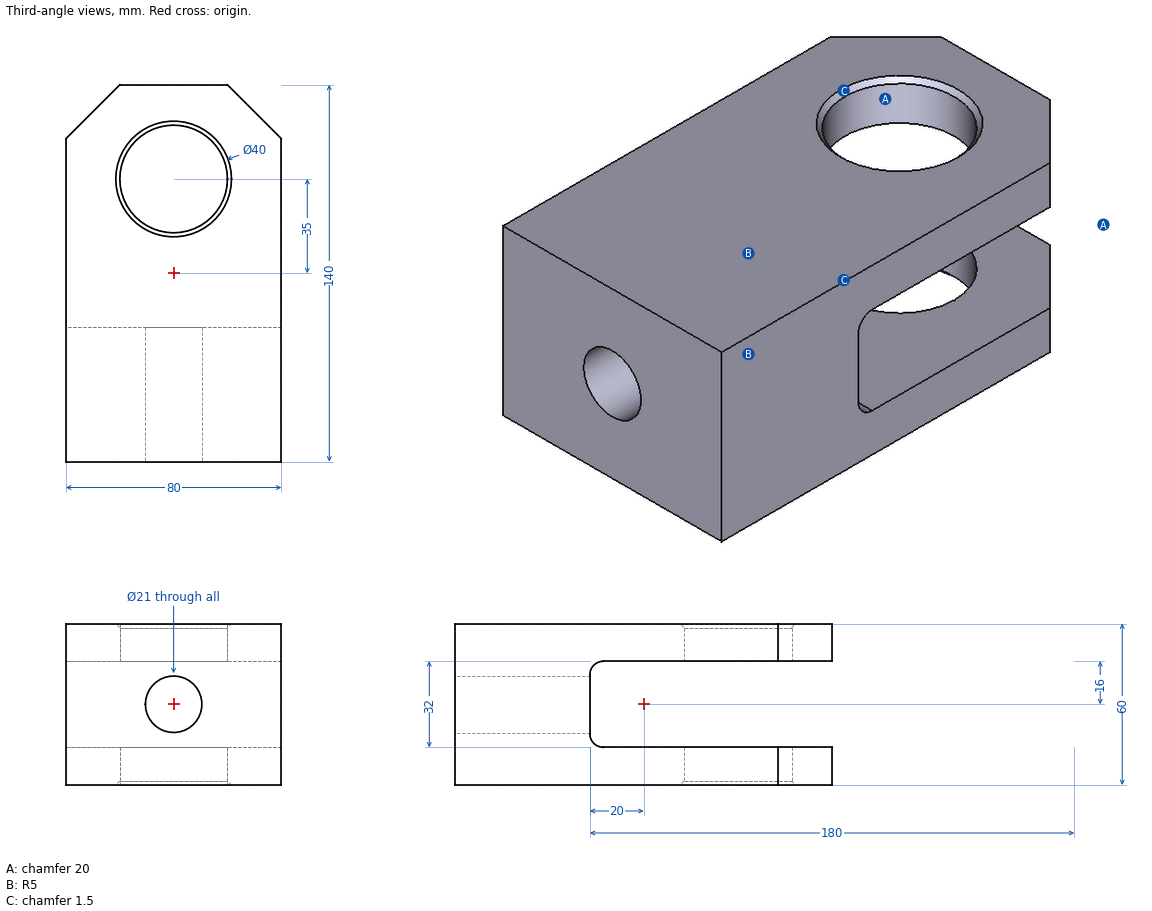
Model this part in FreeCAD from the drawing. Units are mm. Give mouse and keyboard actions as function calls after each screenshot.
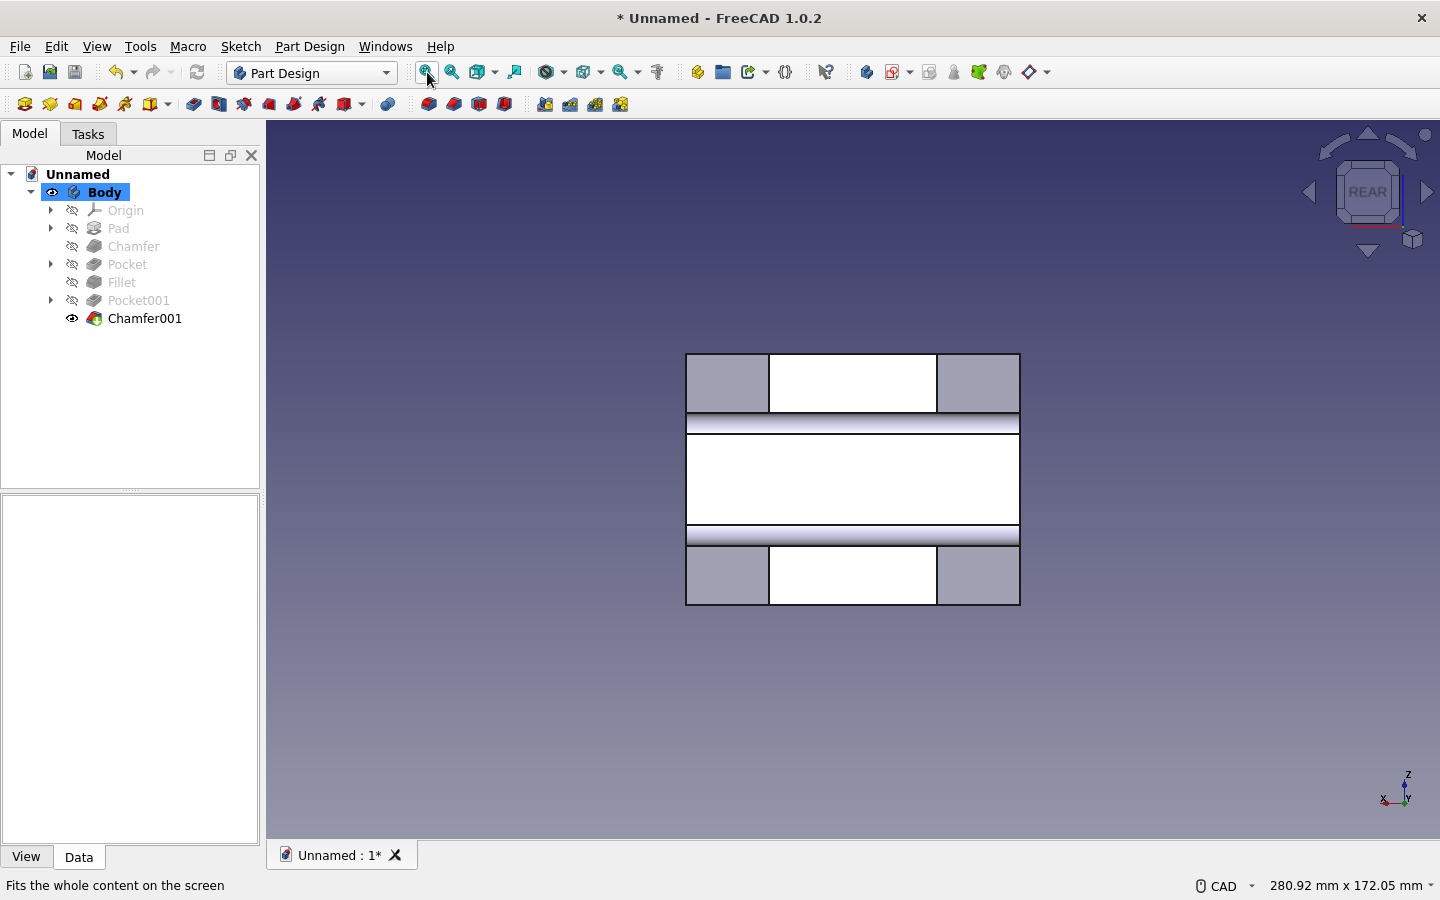
click(757, 479)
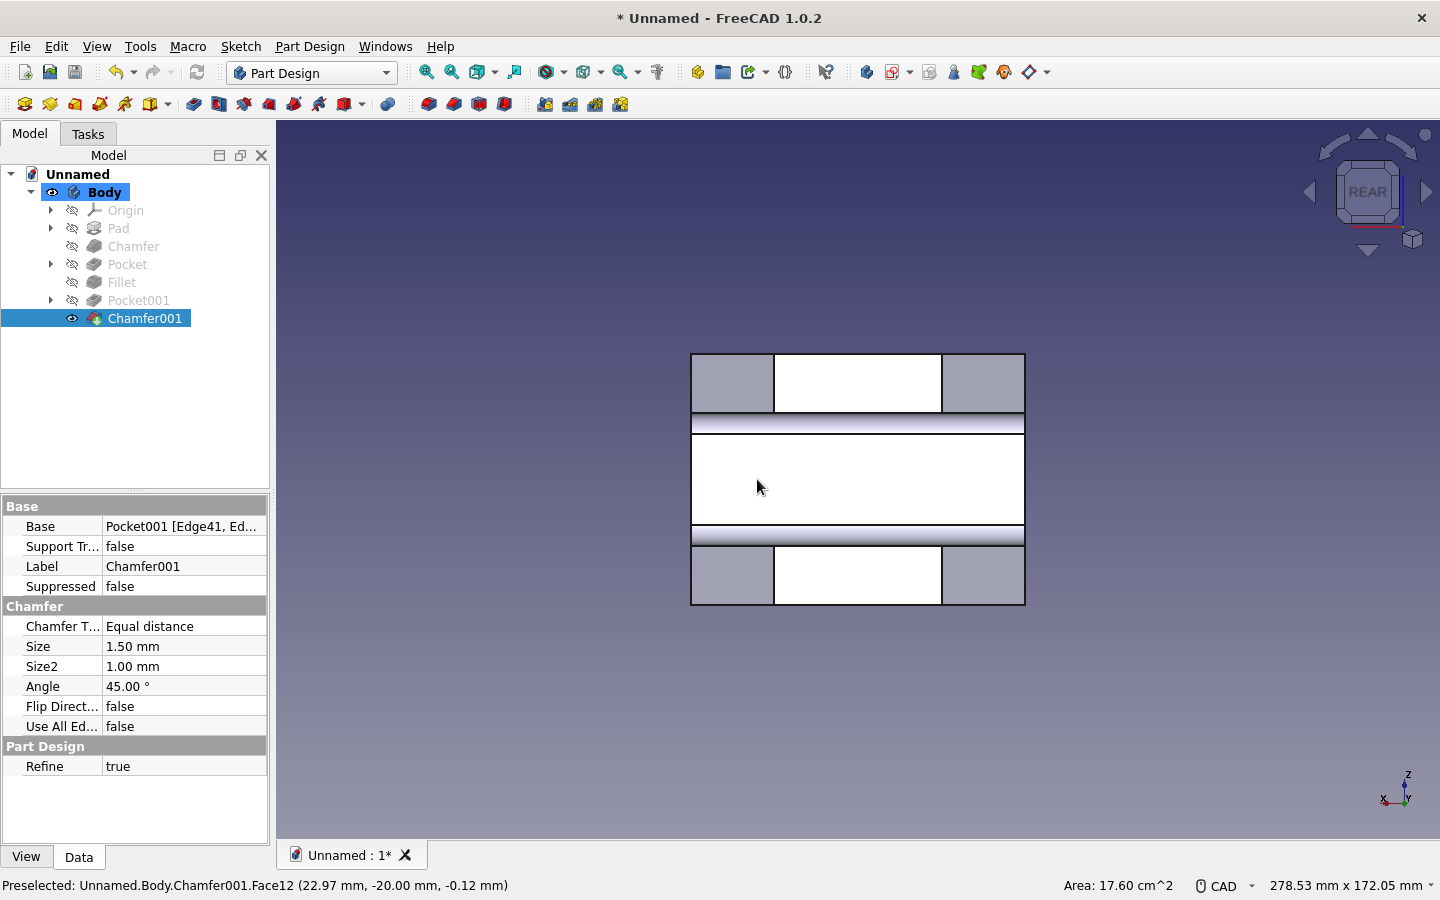
click(892, 72)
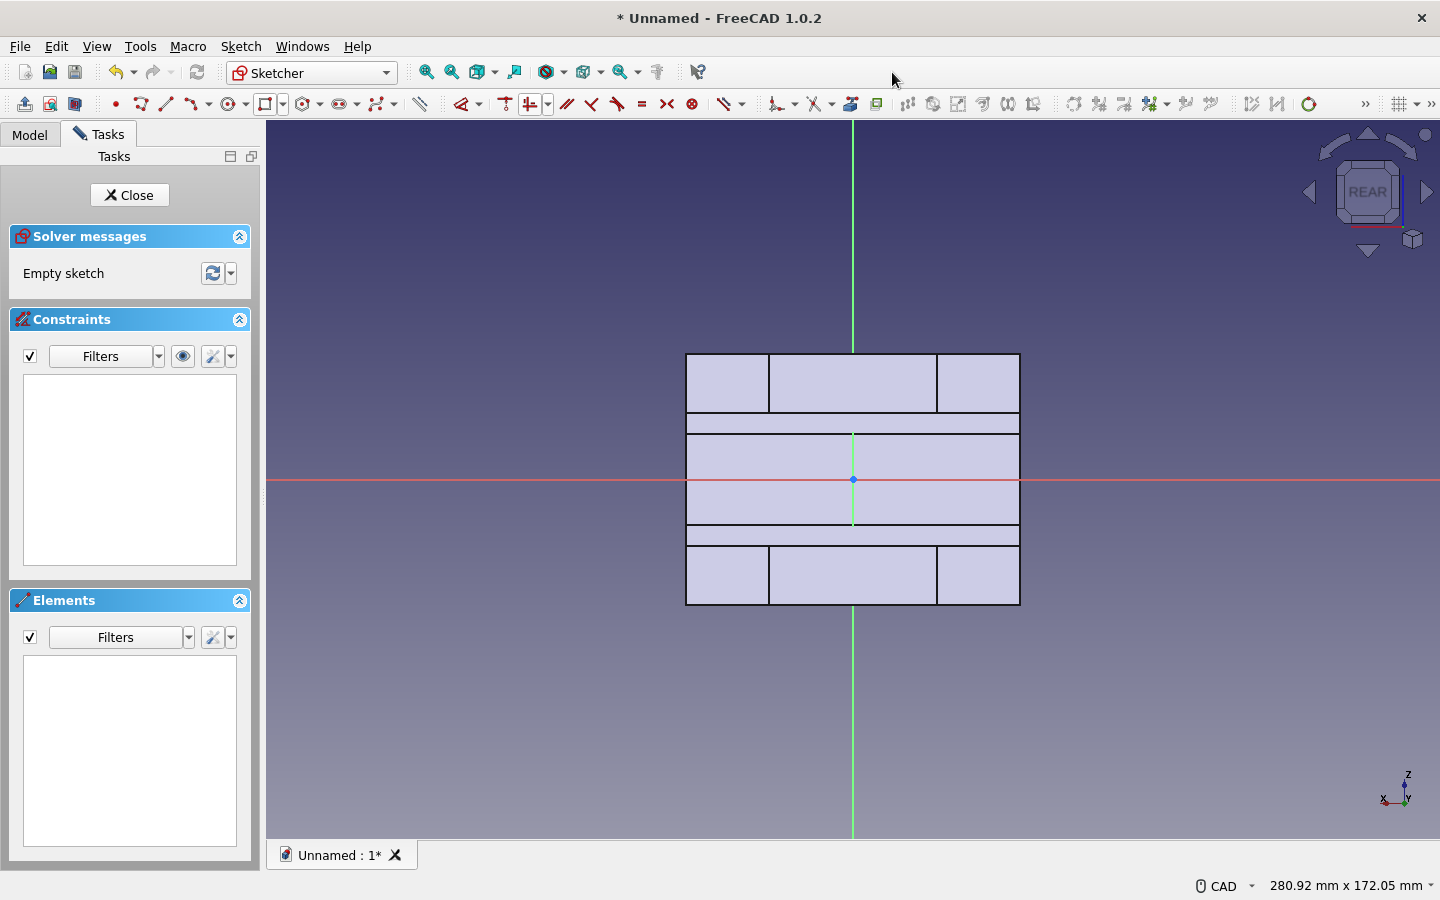
scroll(870, 479, up, 8)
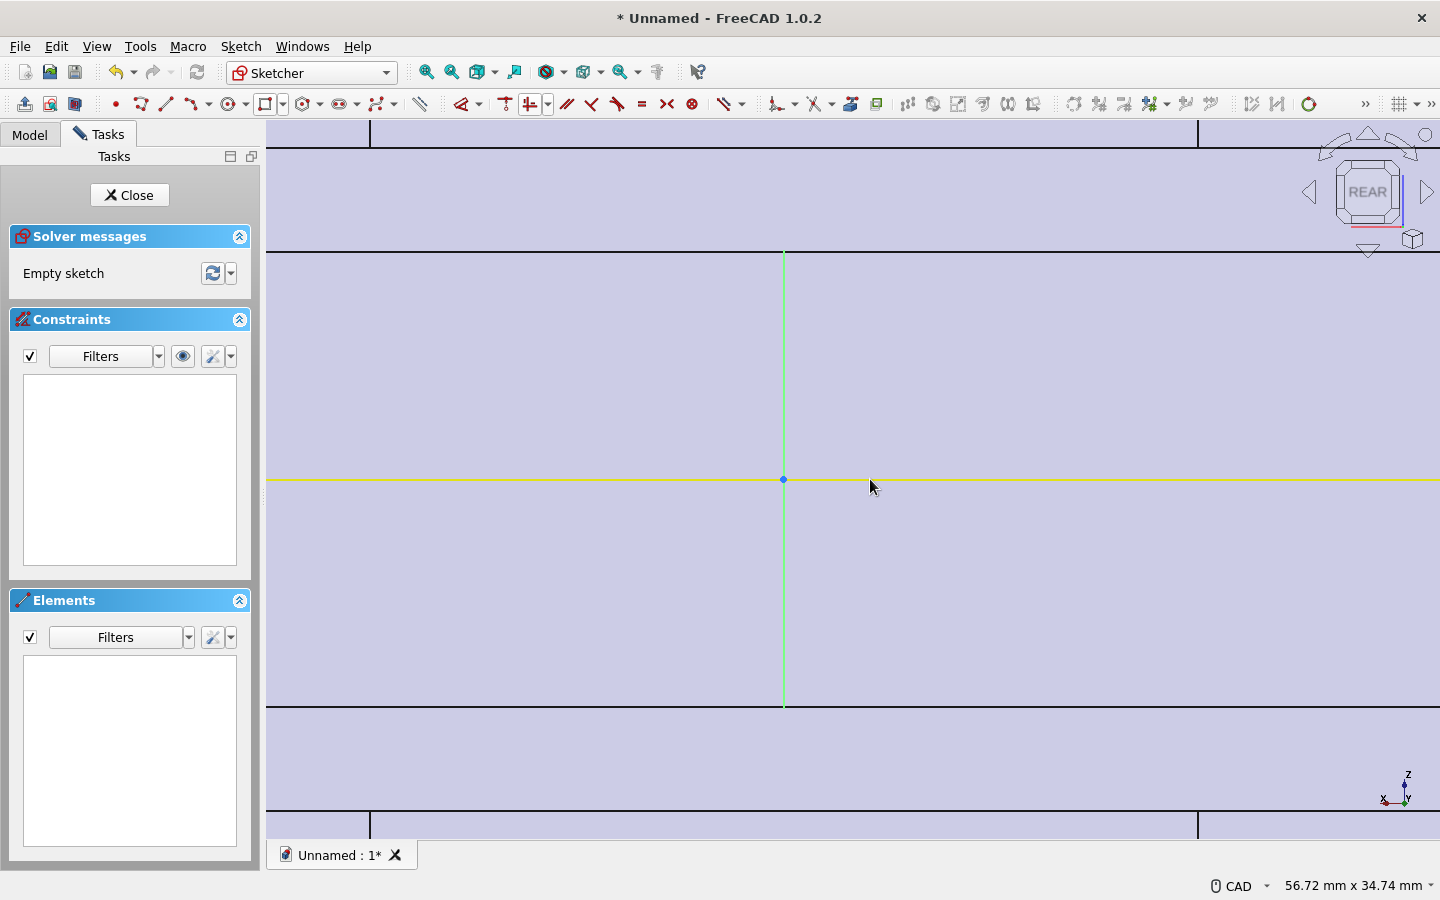
click(228, 104)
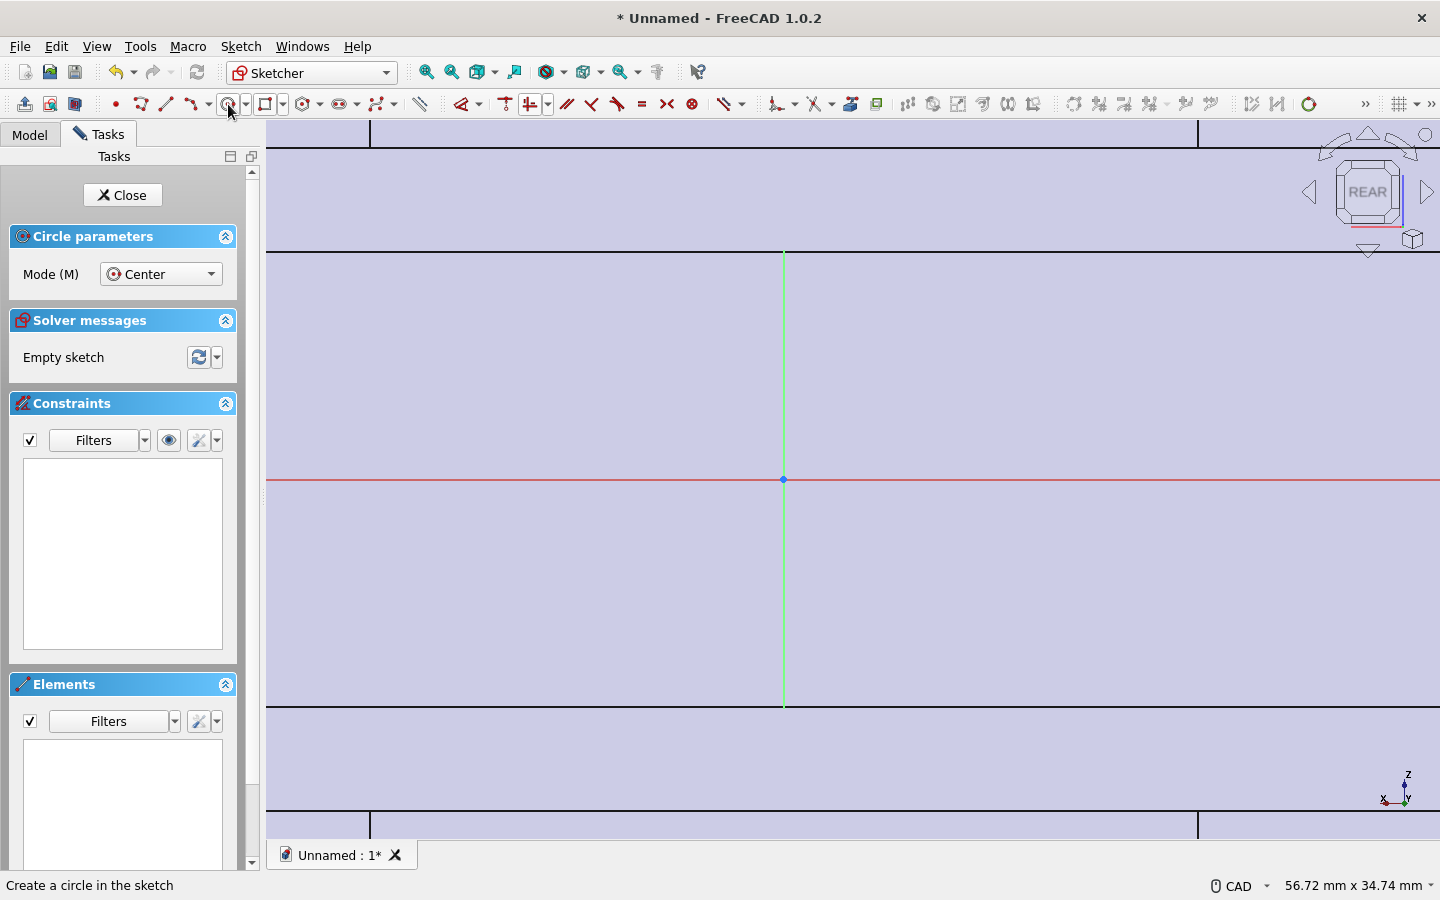
click(784, 480)
move(937, 326)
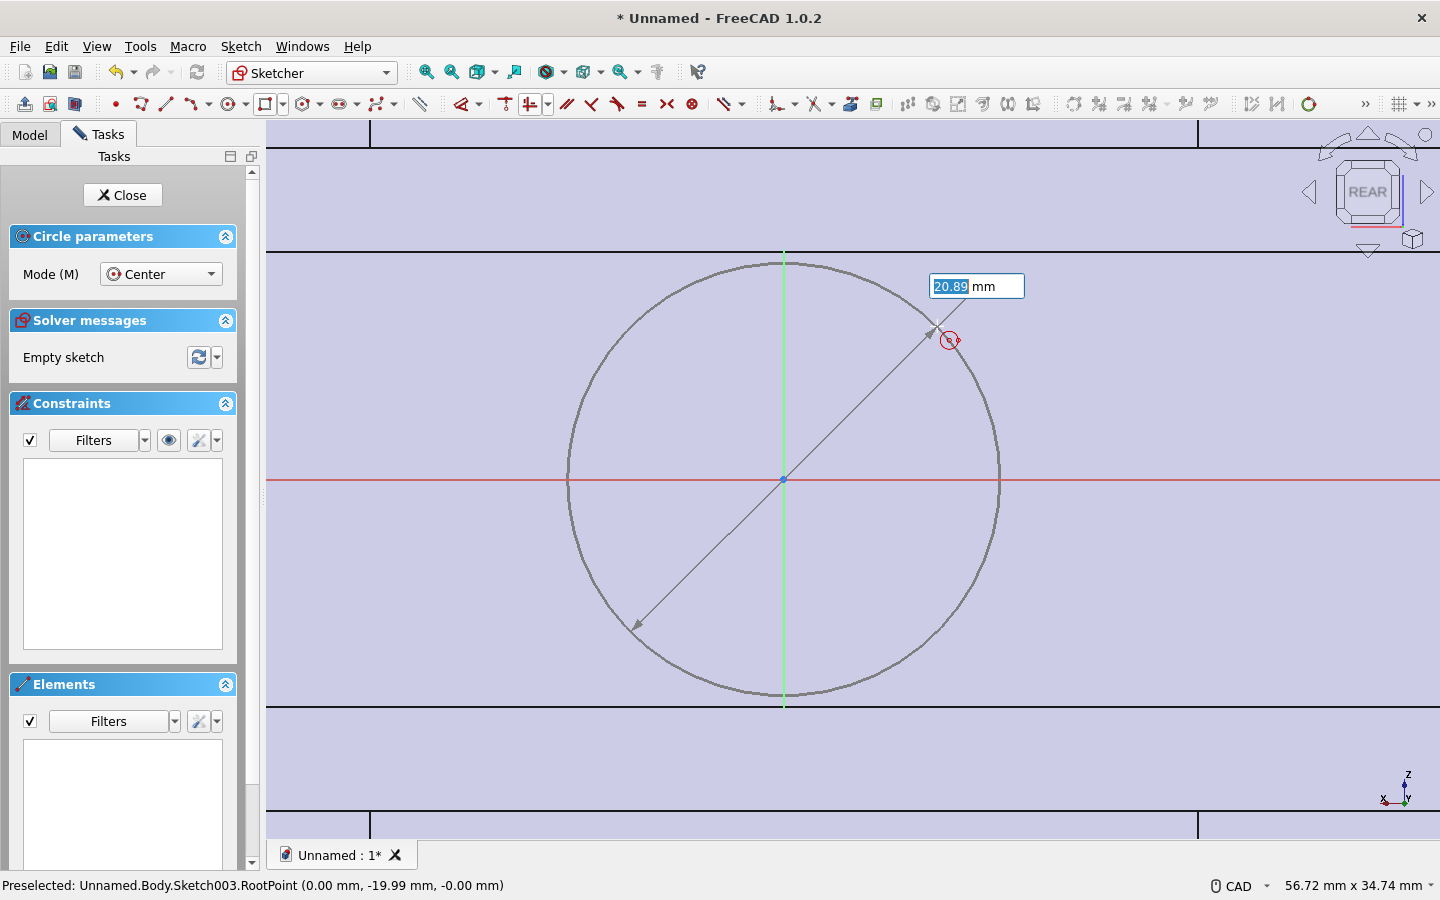
text(21)
key(Return)
key(Escape)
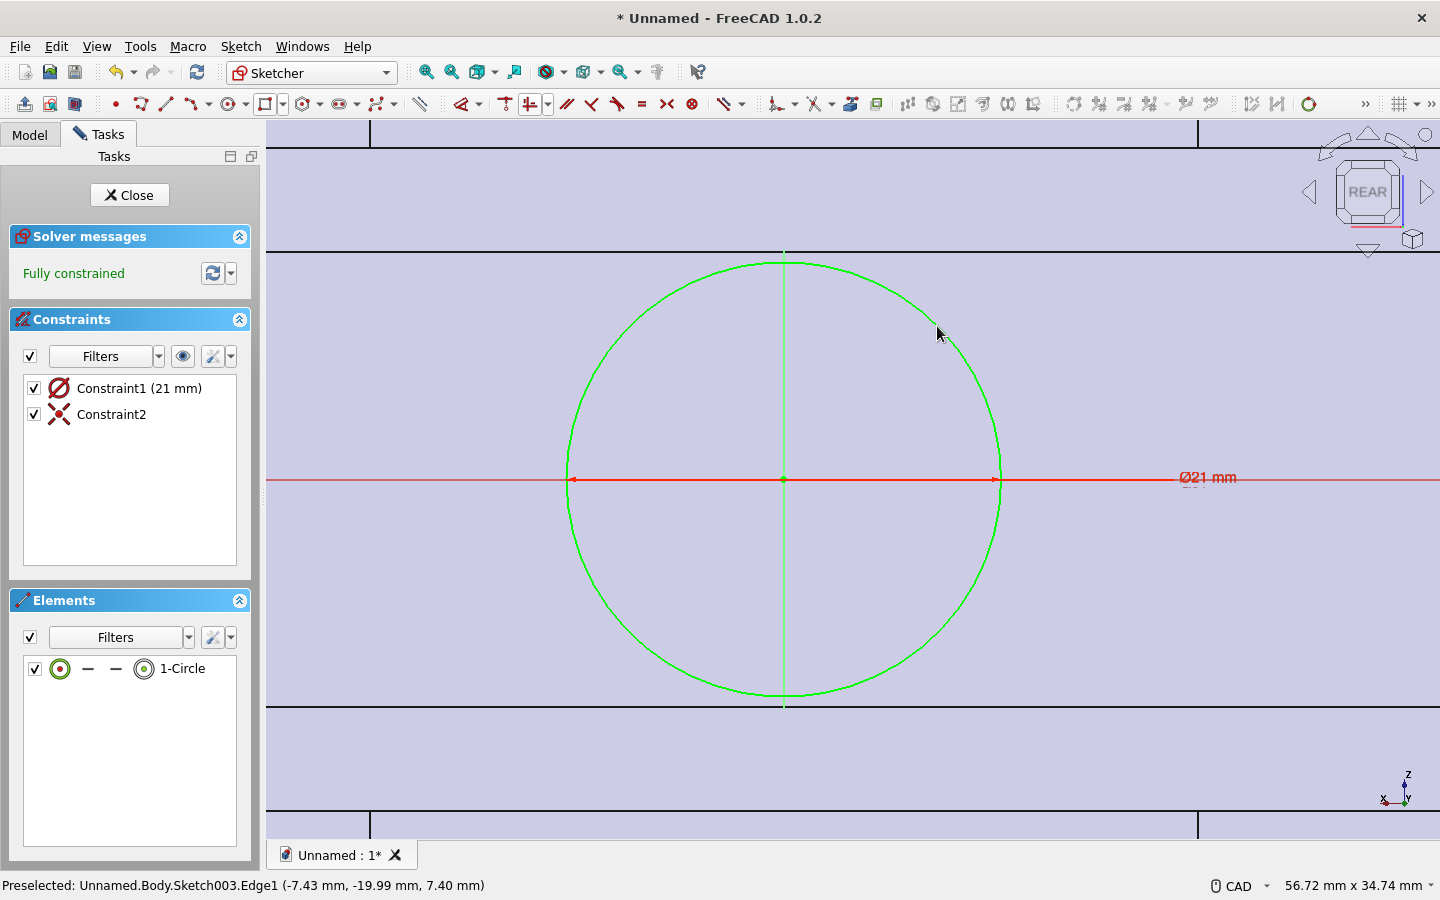
click(130, 195)